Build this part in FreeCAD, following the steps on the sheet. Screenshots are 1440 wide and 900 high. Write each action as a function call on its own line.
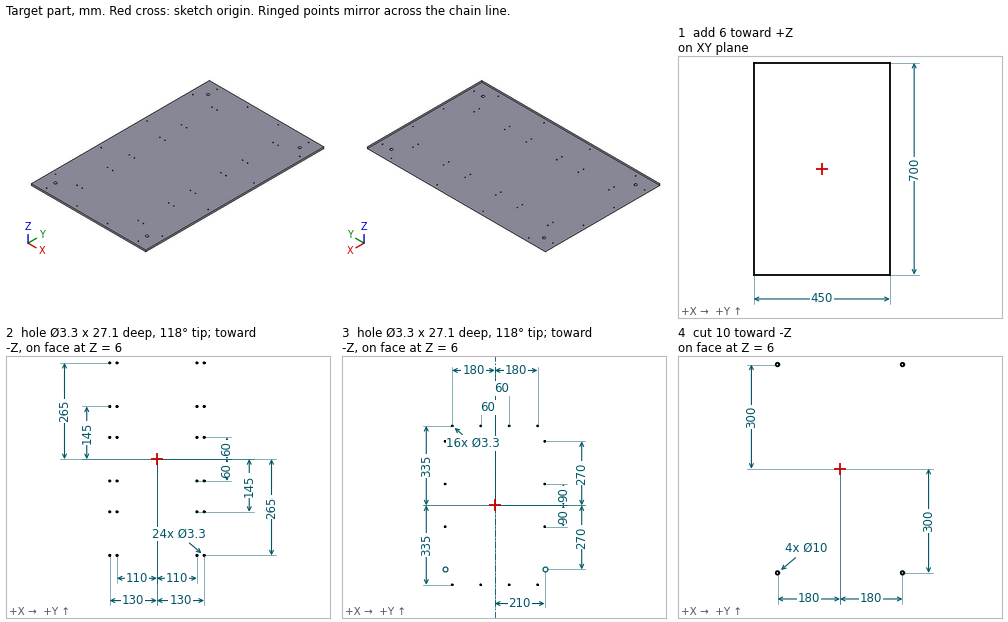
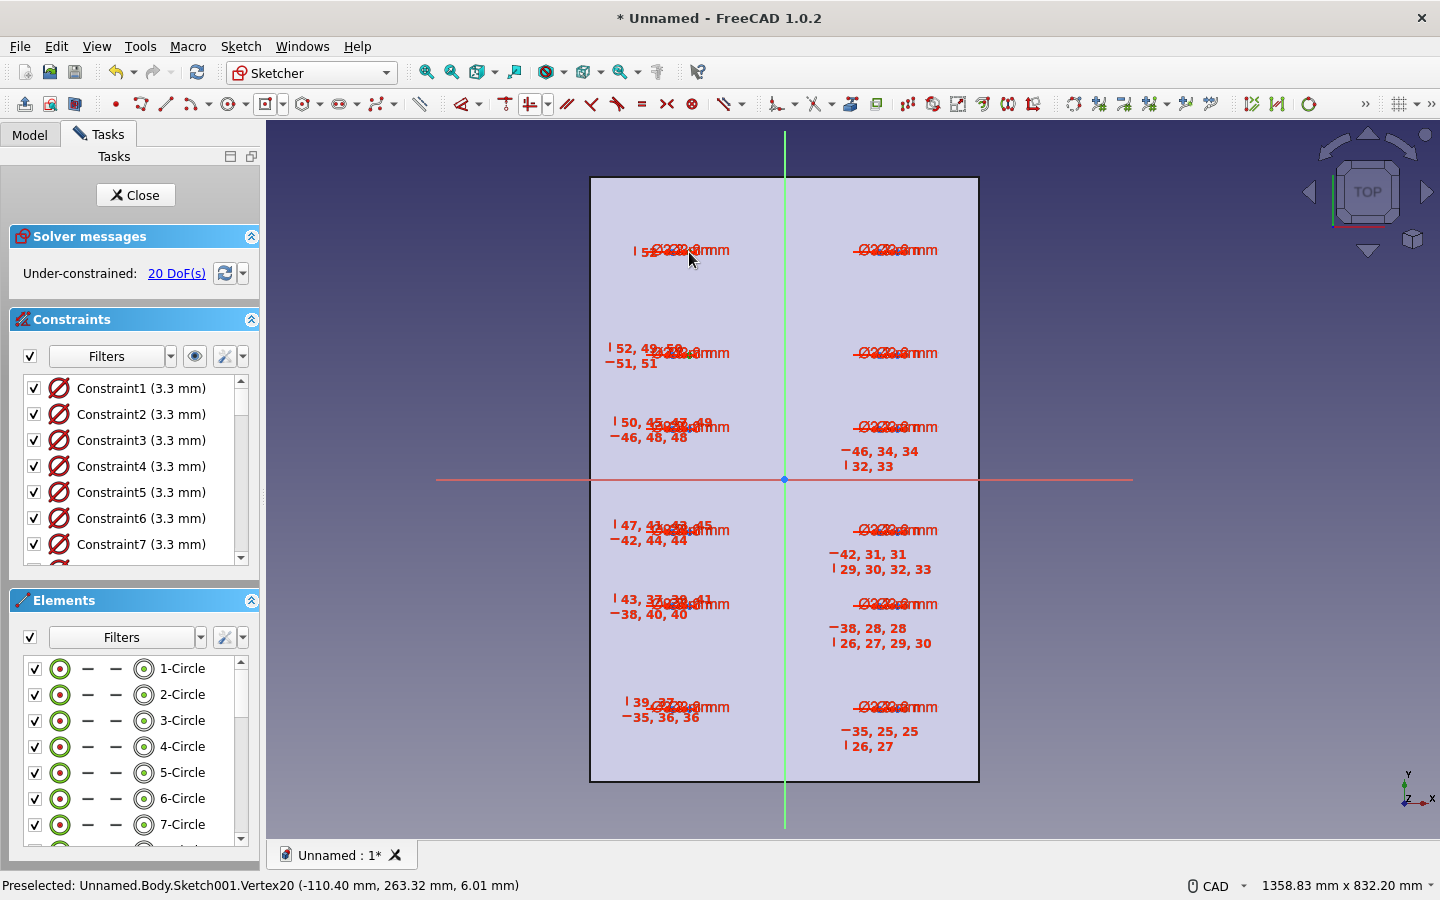
click(548, 104)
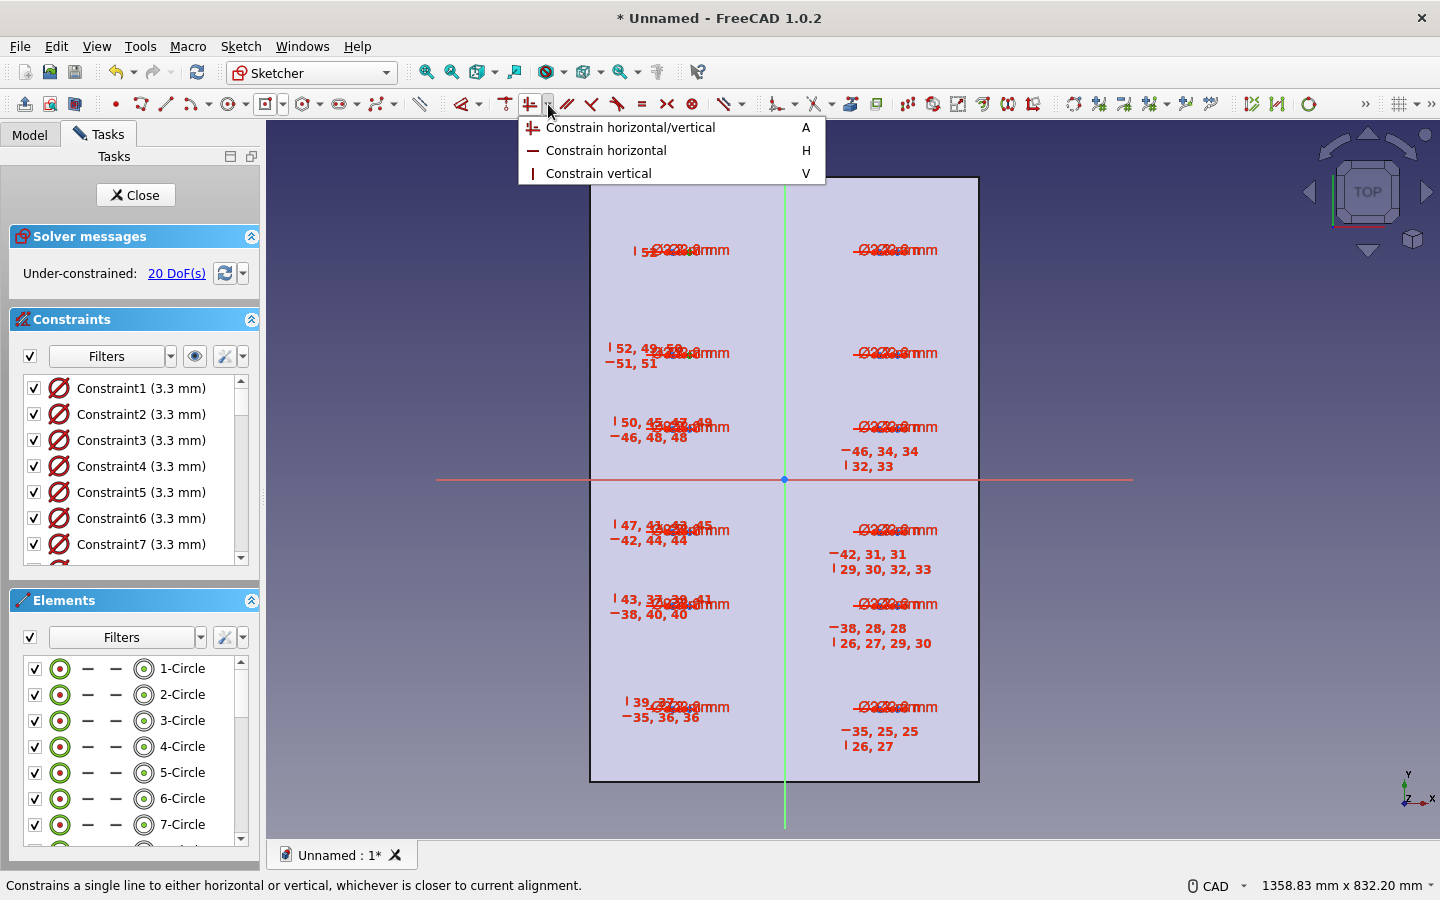
click(672, 174)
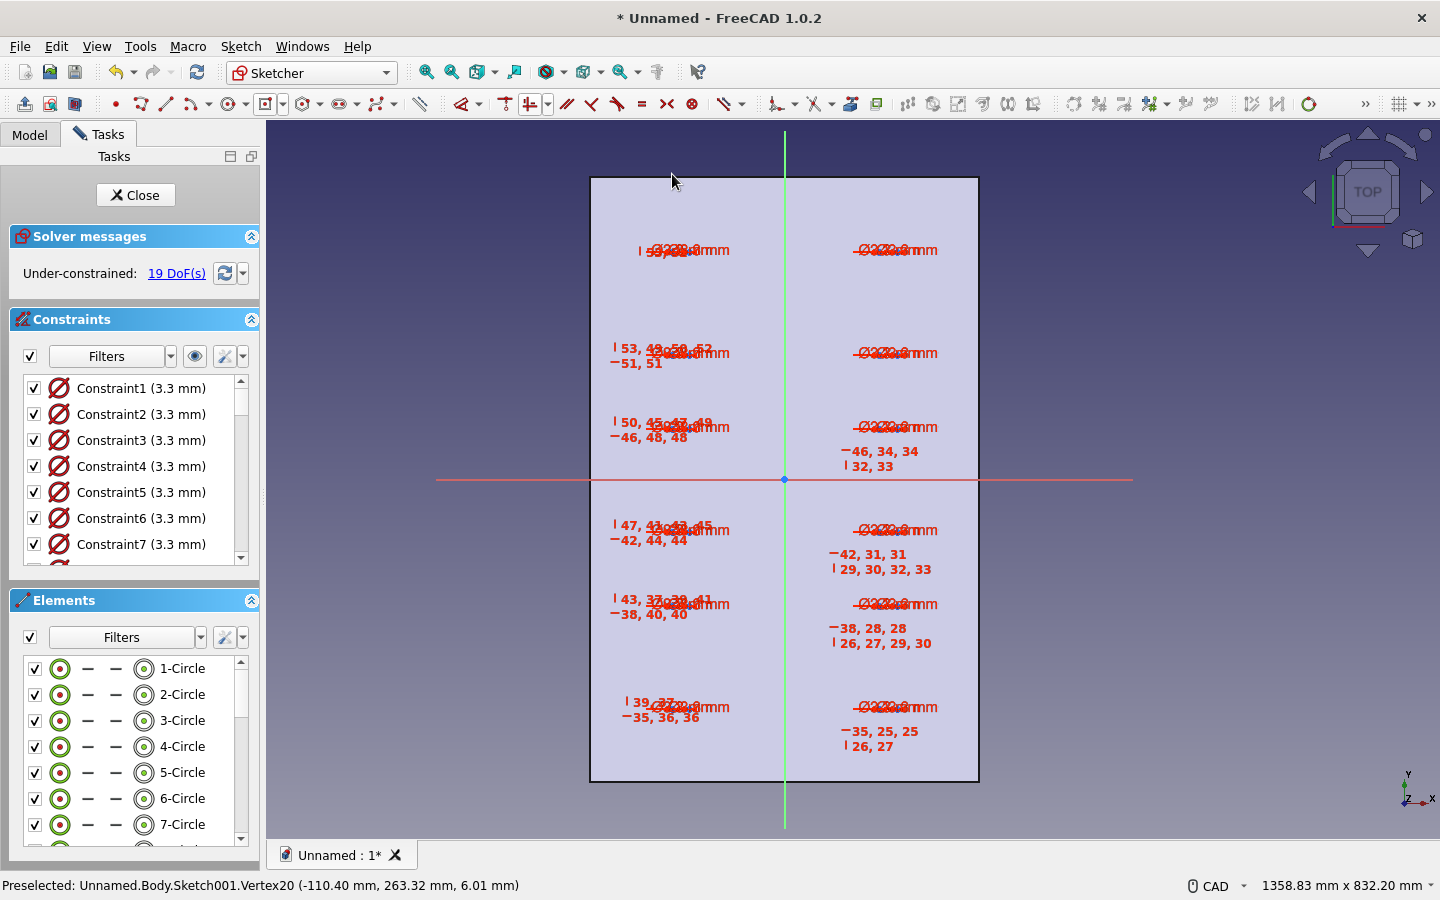
scroll(672, 252, up, 4)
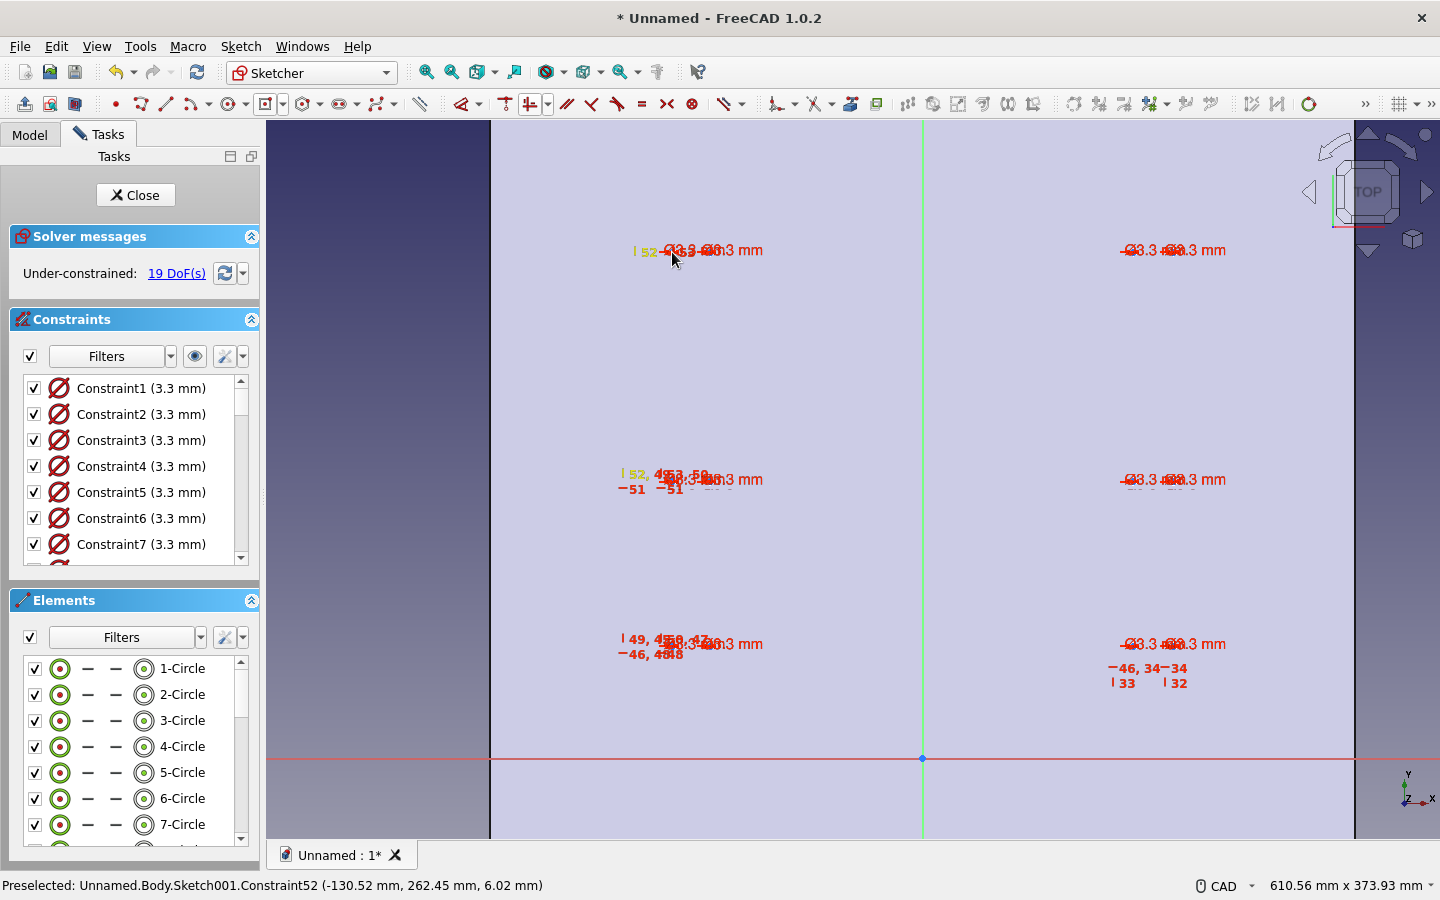
scroll(672, 252, up, 4)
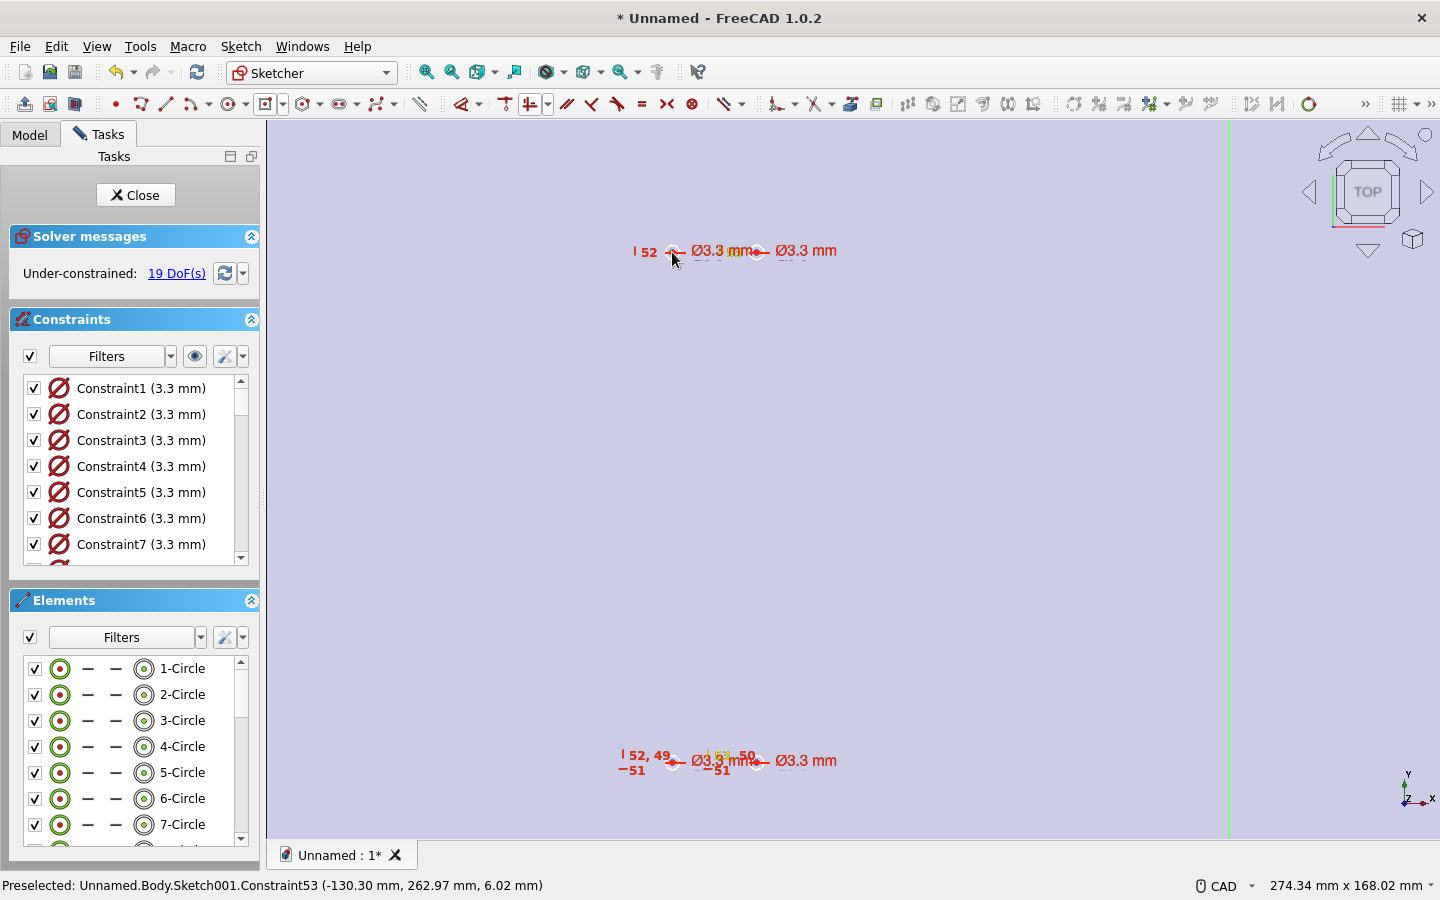
click(673, 253)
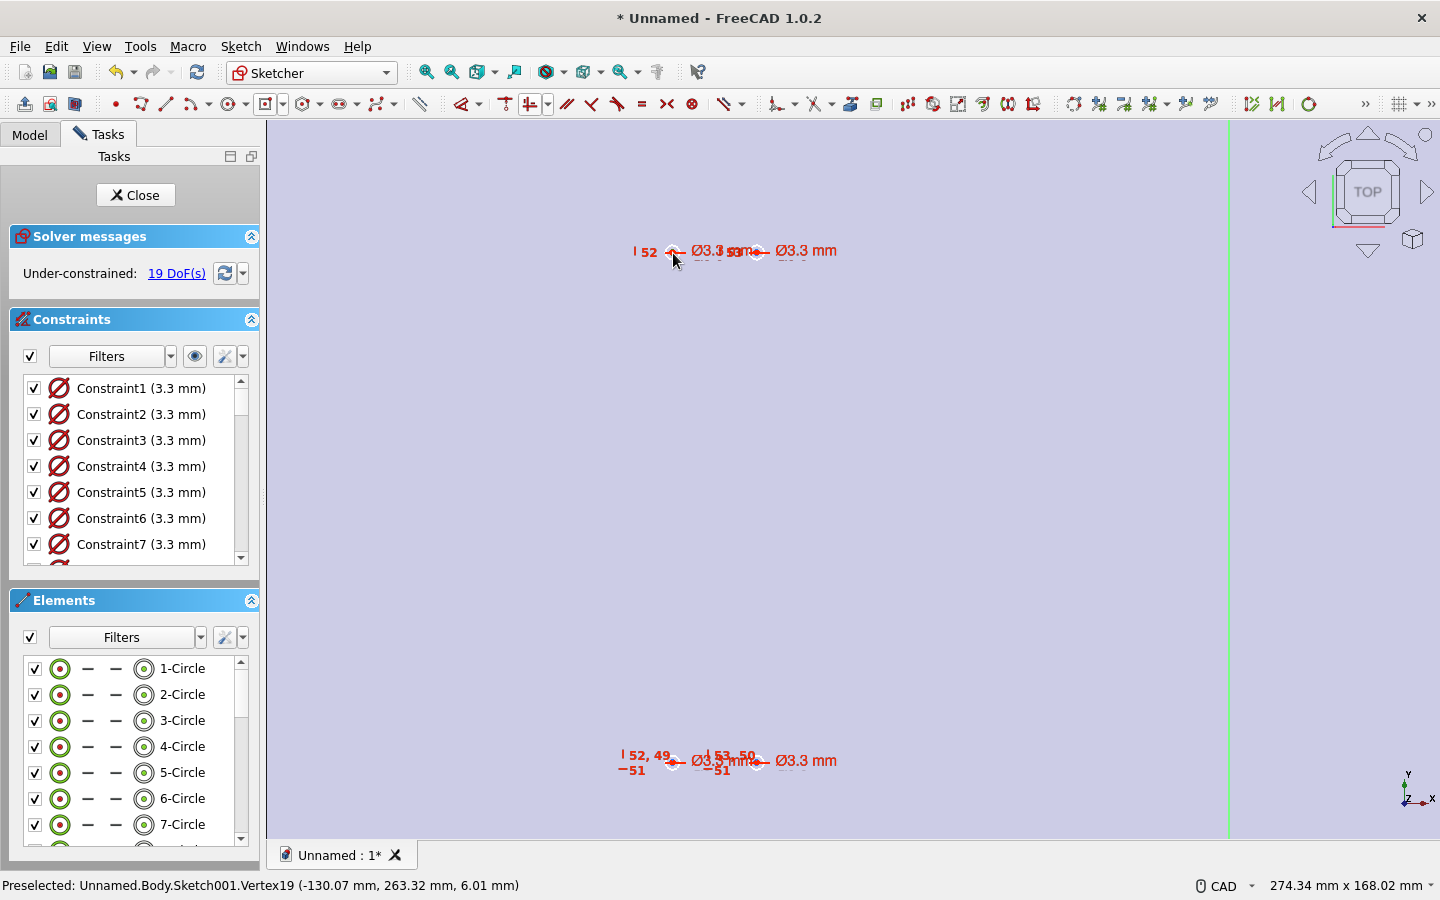
scroll(672, 252, down, 8)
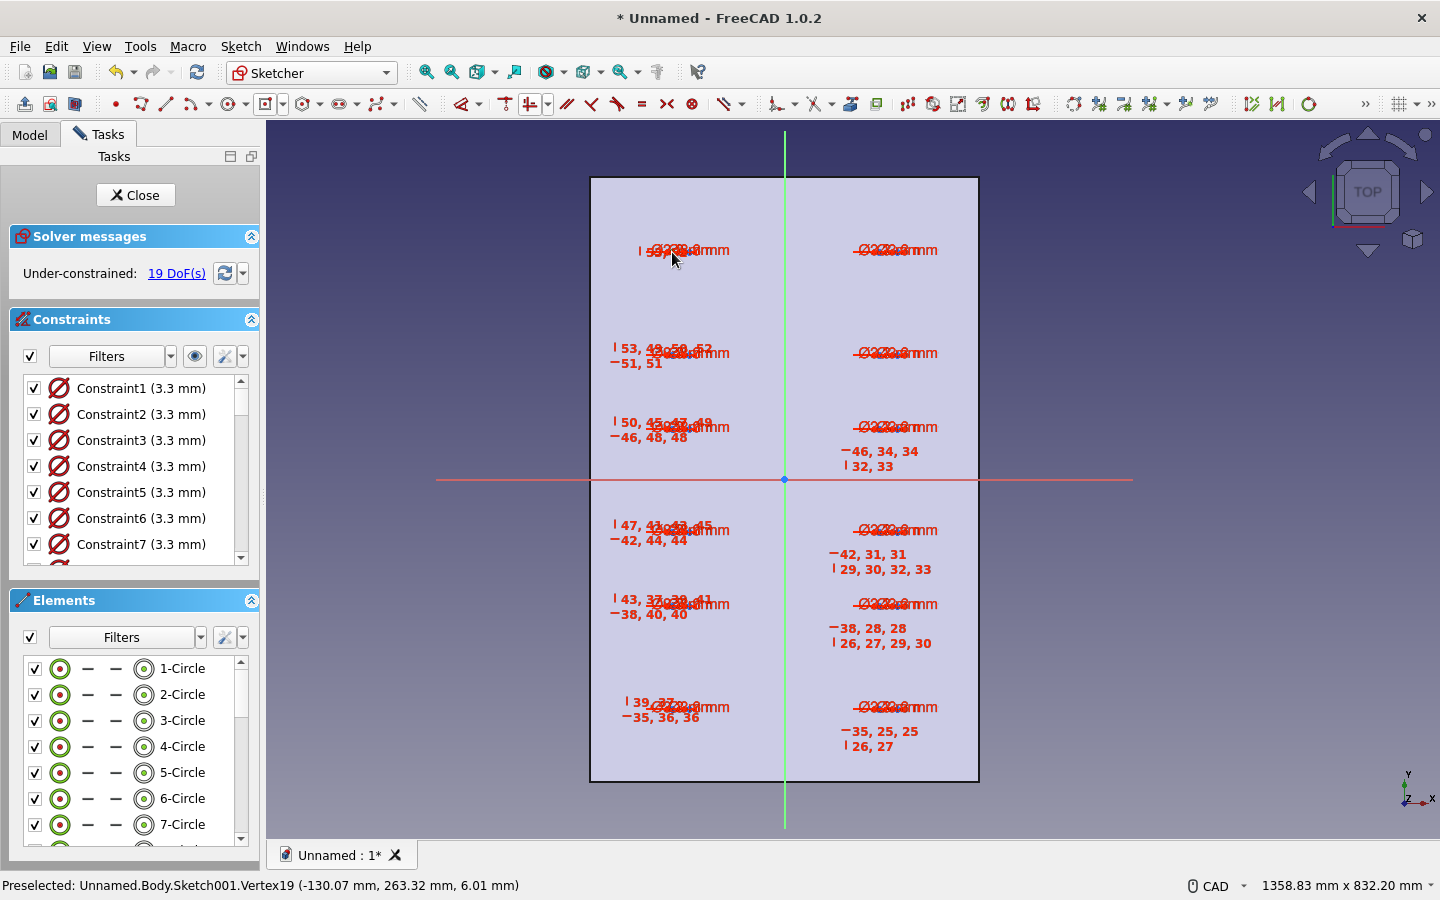
click(689, 252)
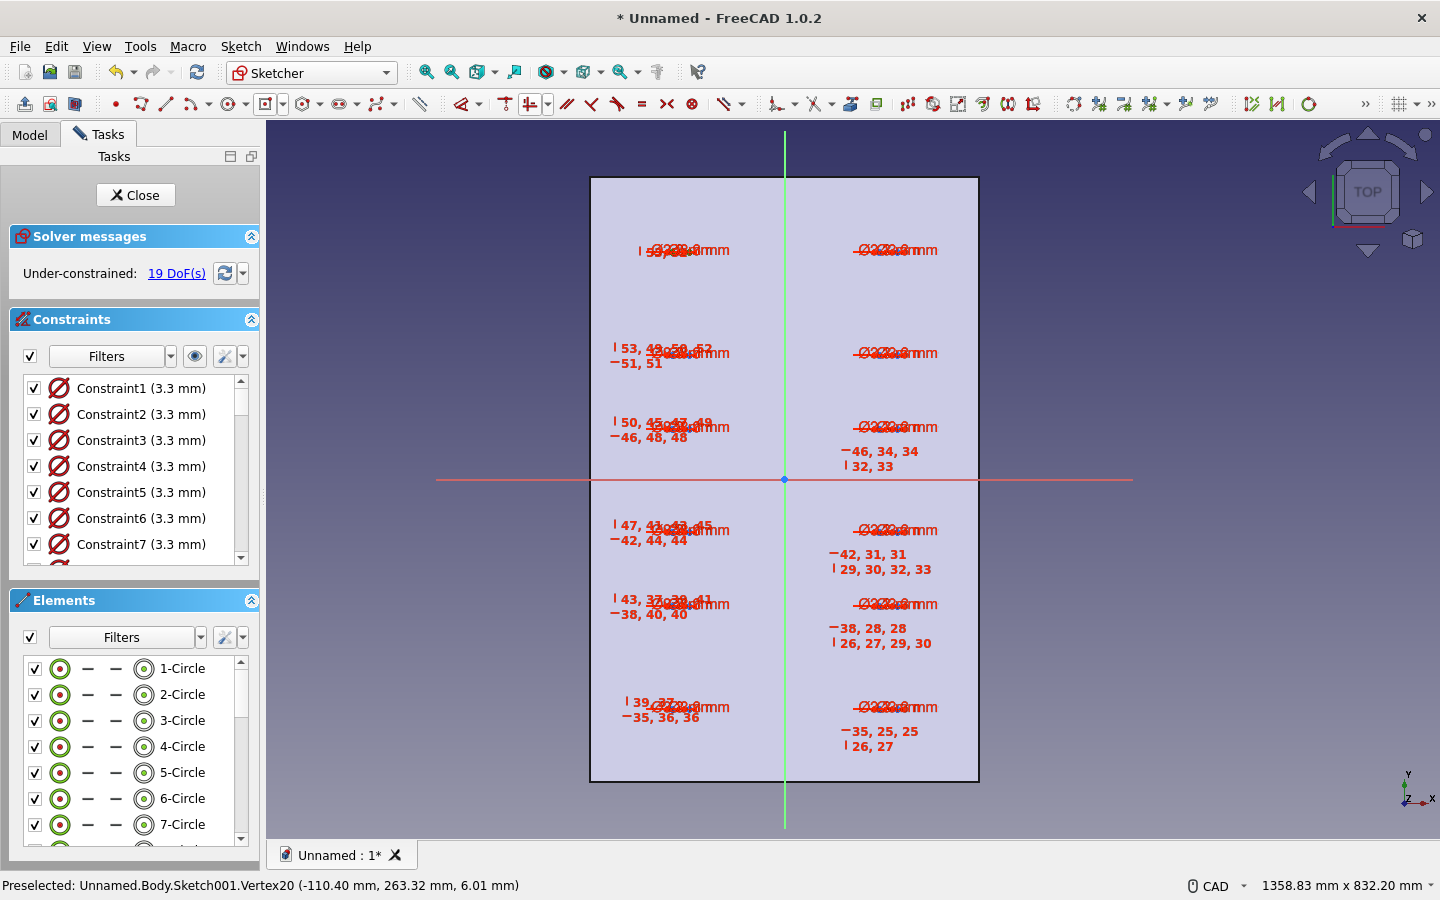
click(548, 104)